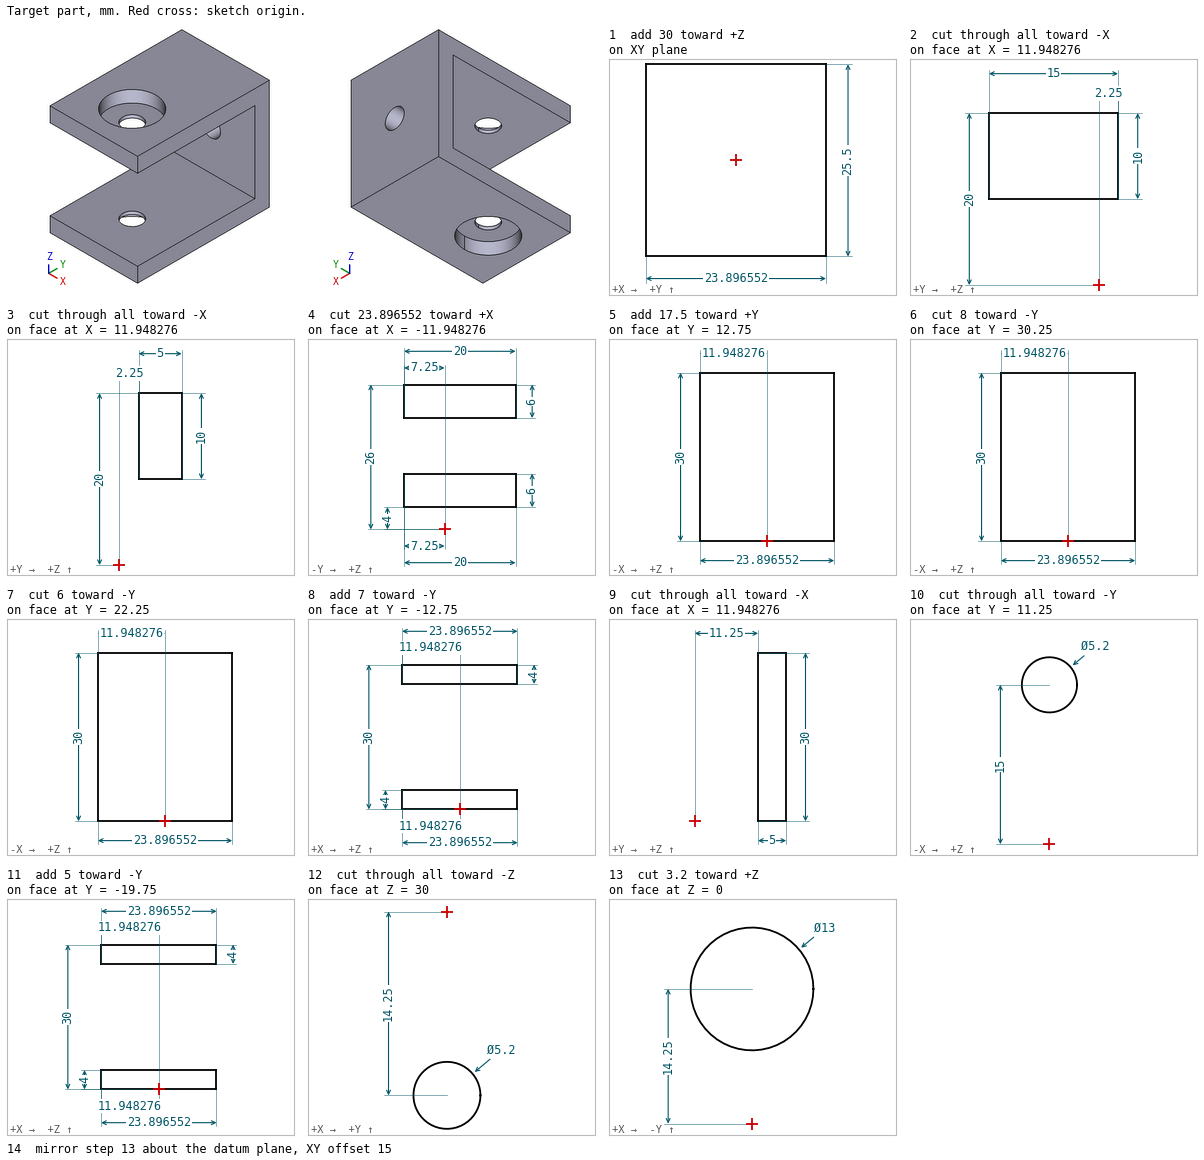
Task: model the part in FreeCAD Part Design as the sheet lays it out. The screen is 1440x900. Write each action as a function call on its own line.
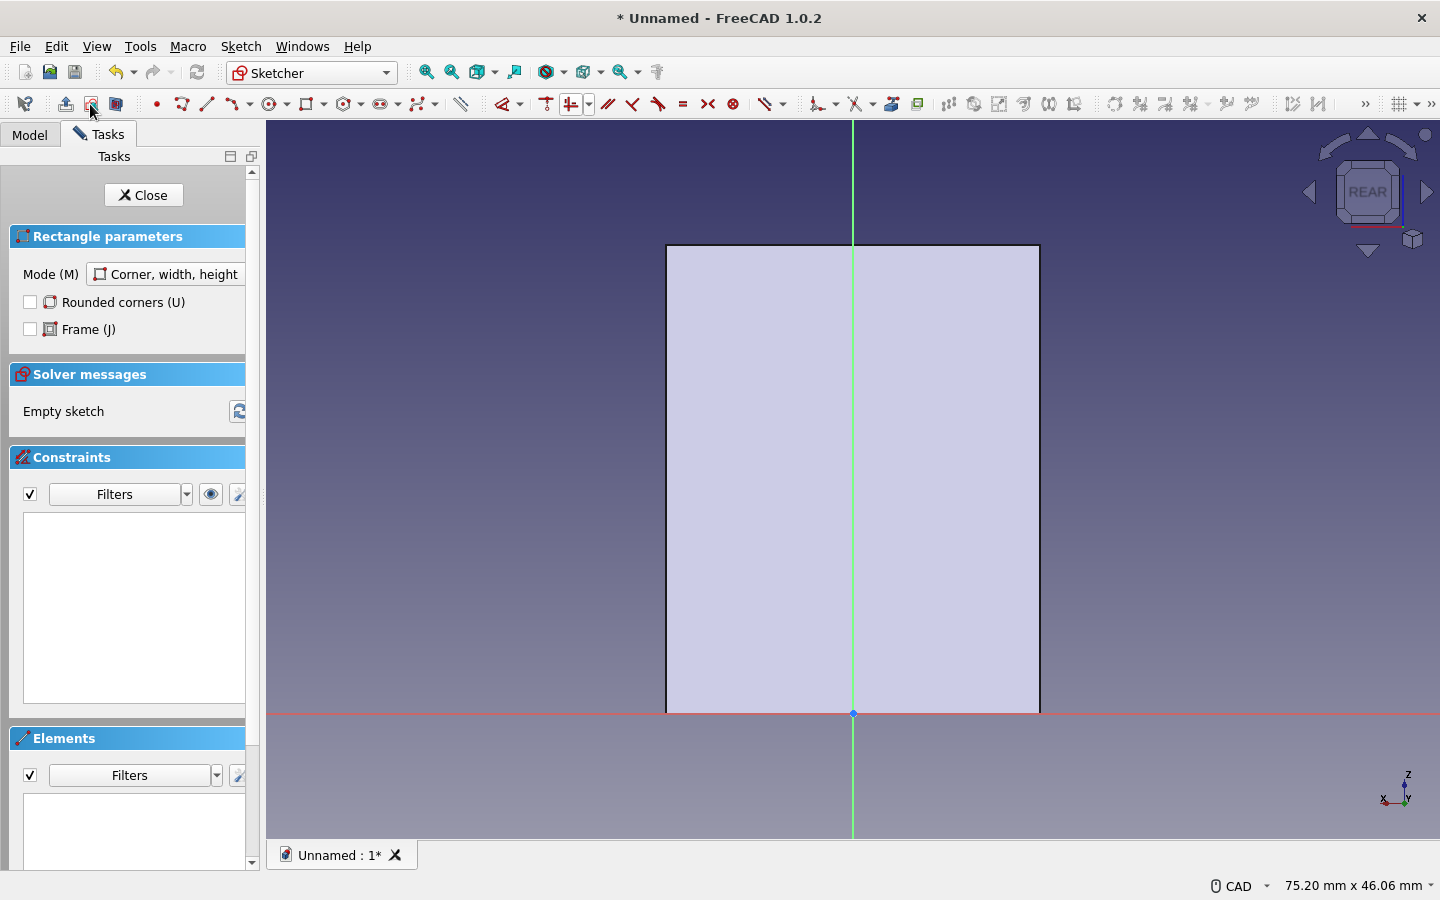
click(666, 245)
click(1040, 714)
key(Escape)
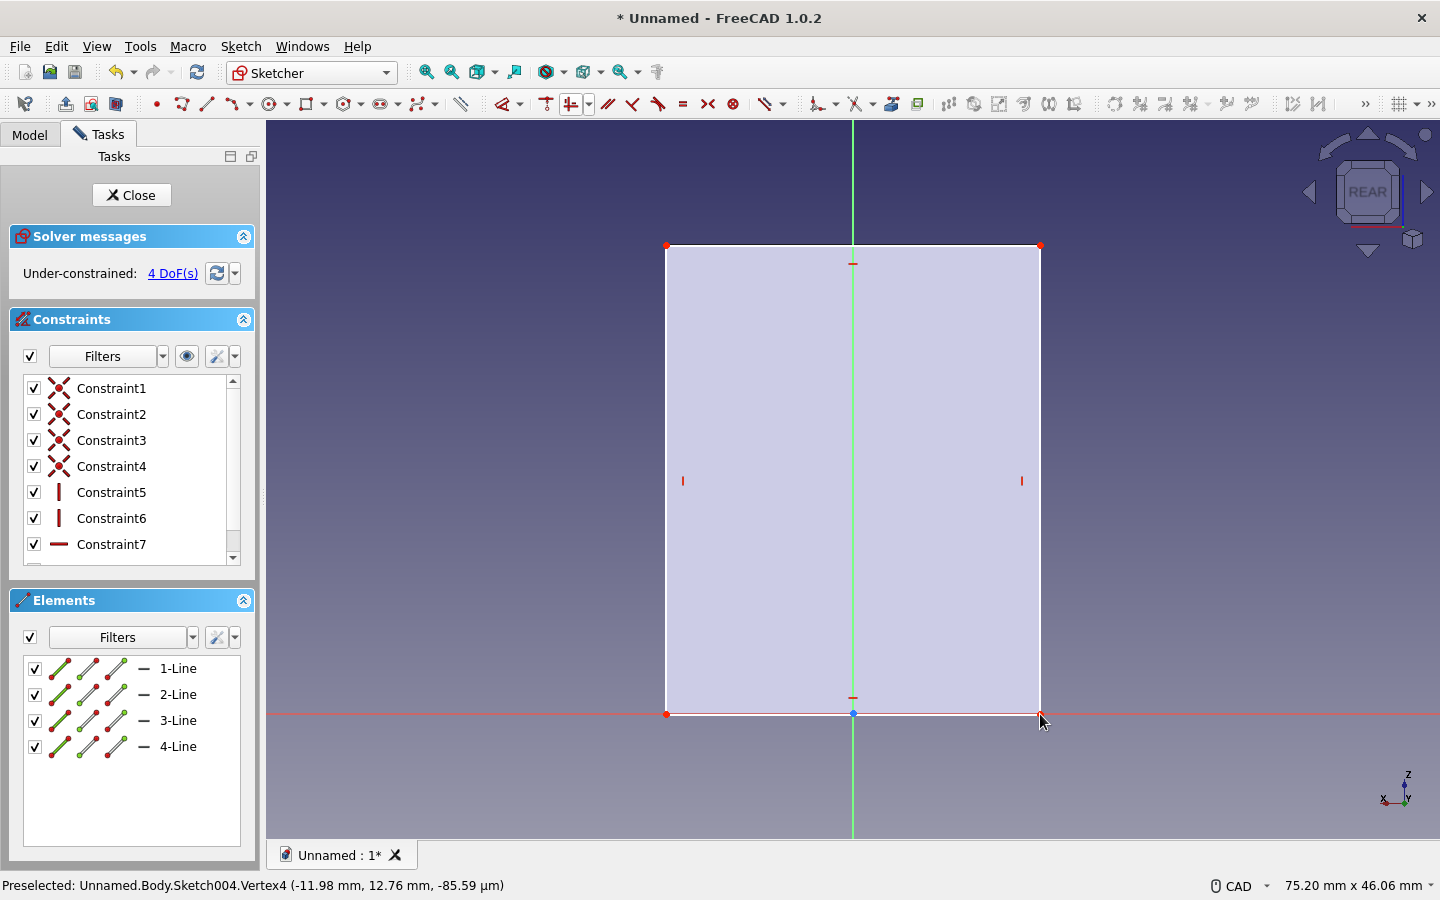
click(666, 715)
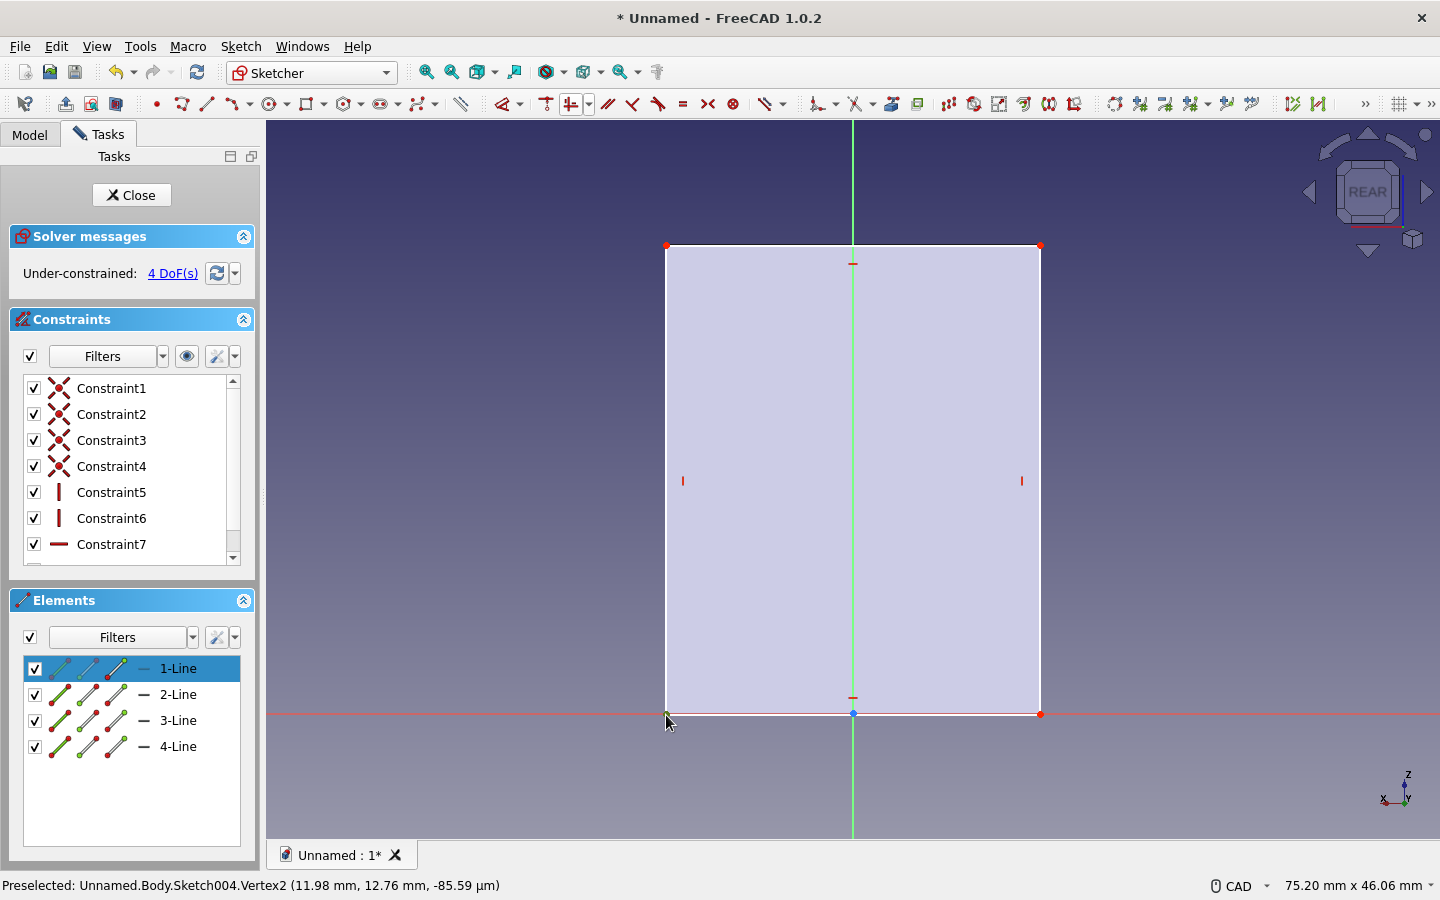
click(364, 714)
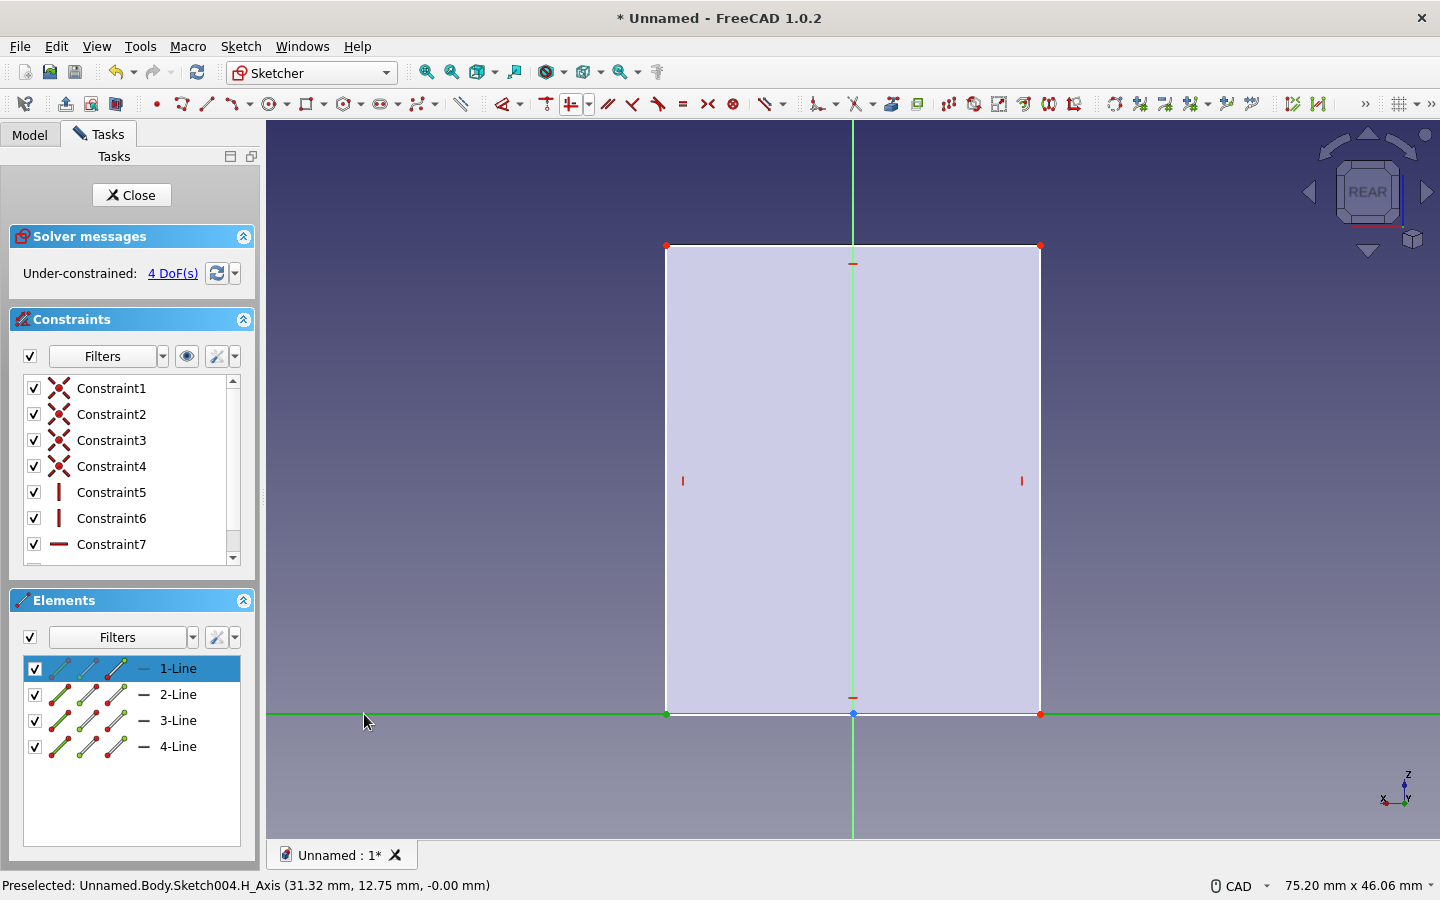
click(546, 104)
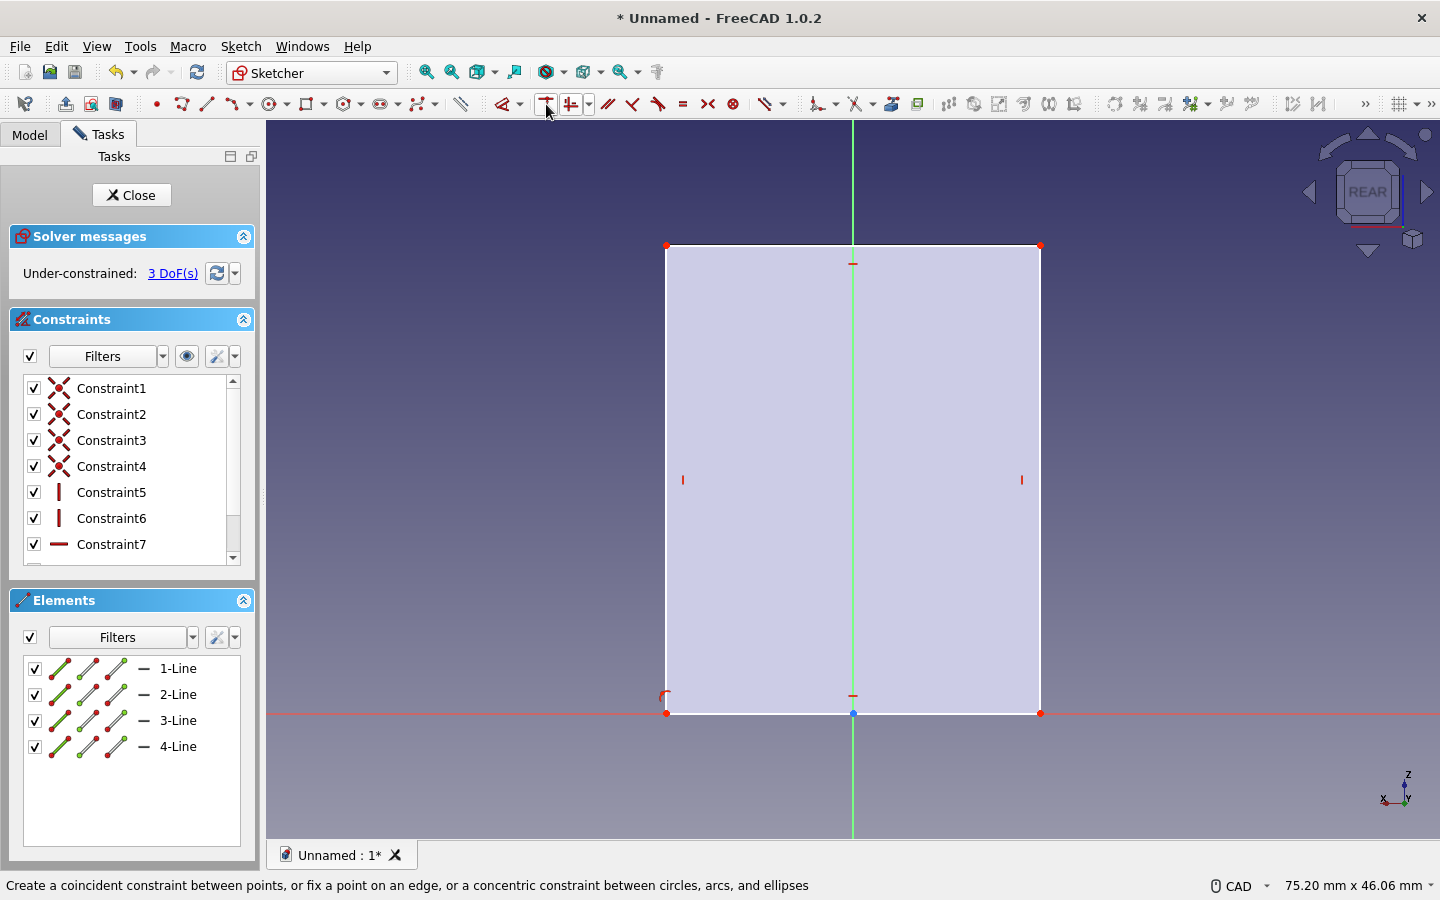
click(502, 104)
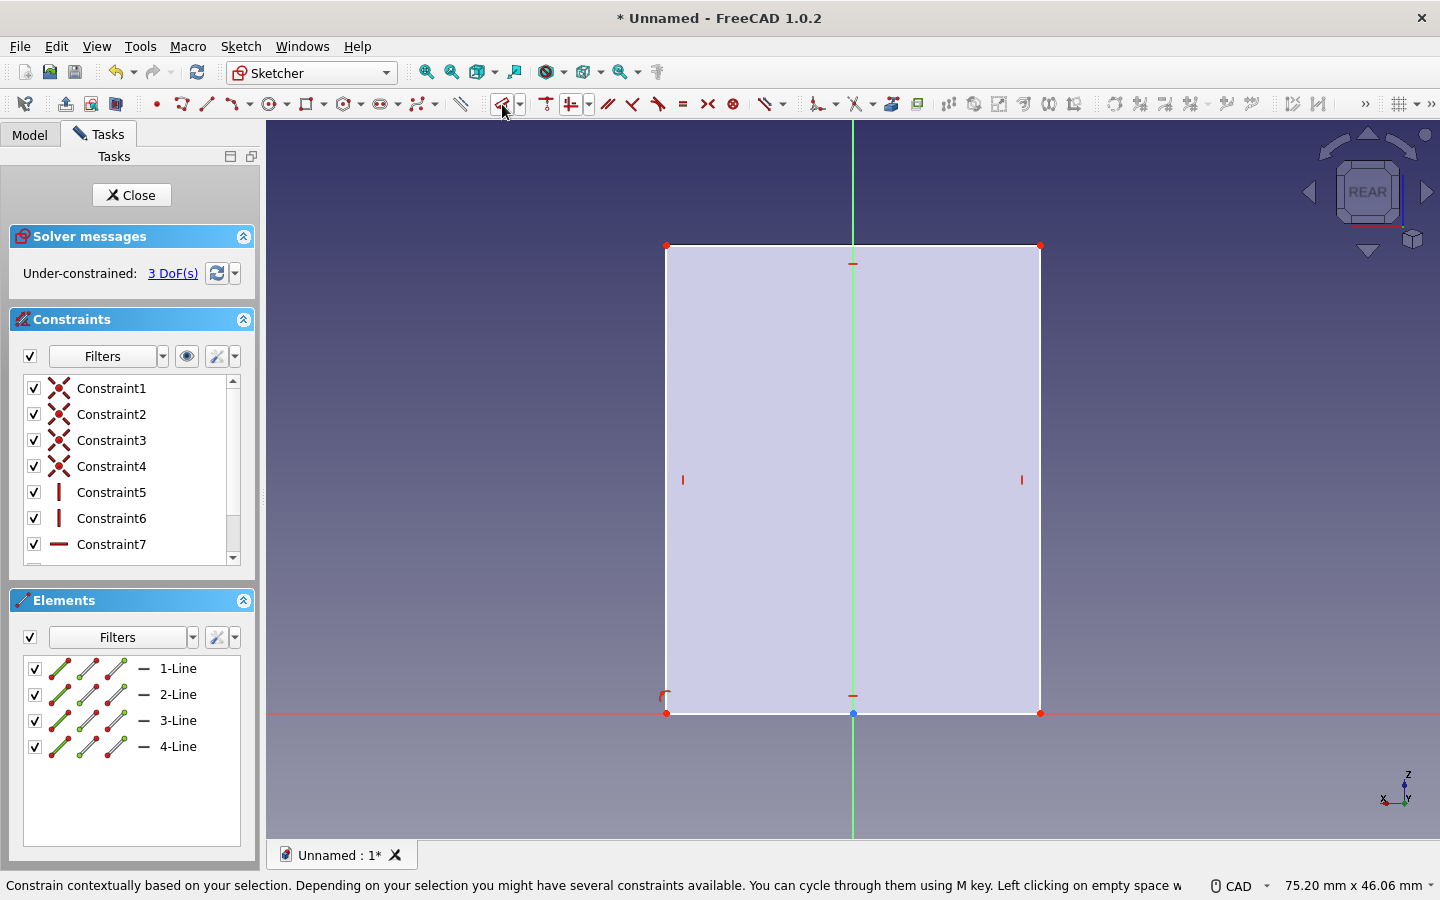
click(666, 386)
click(632, 480)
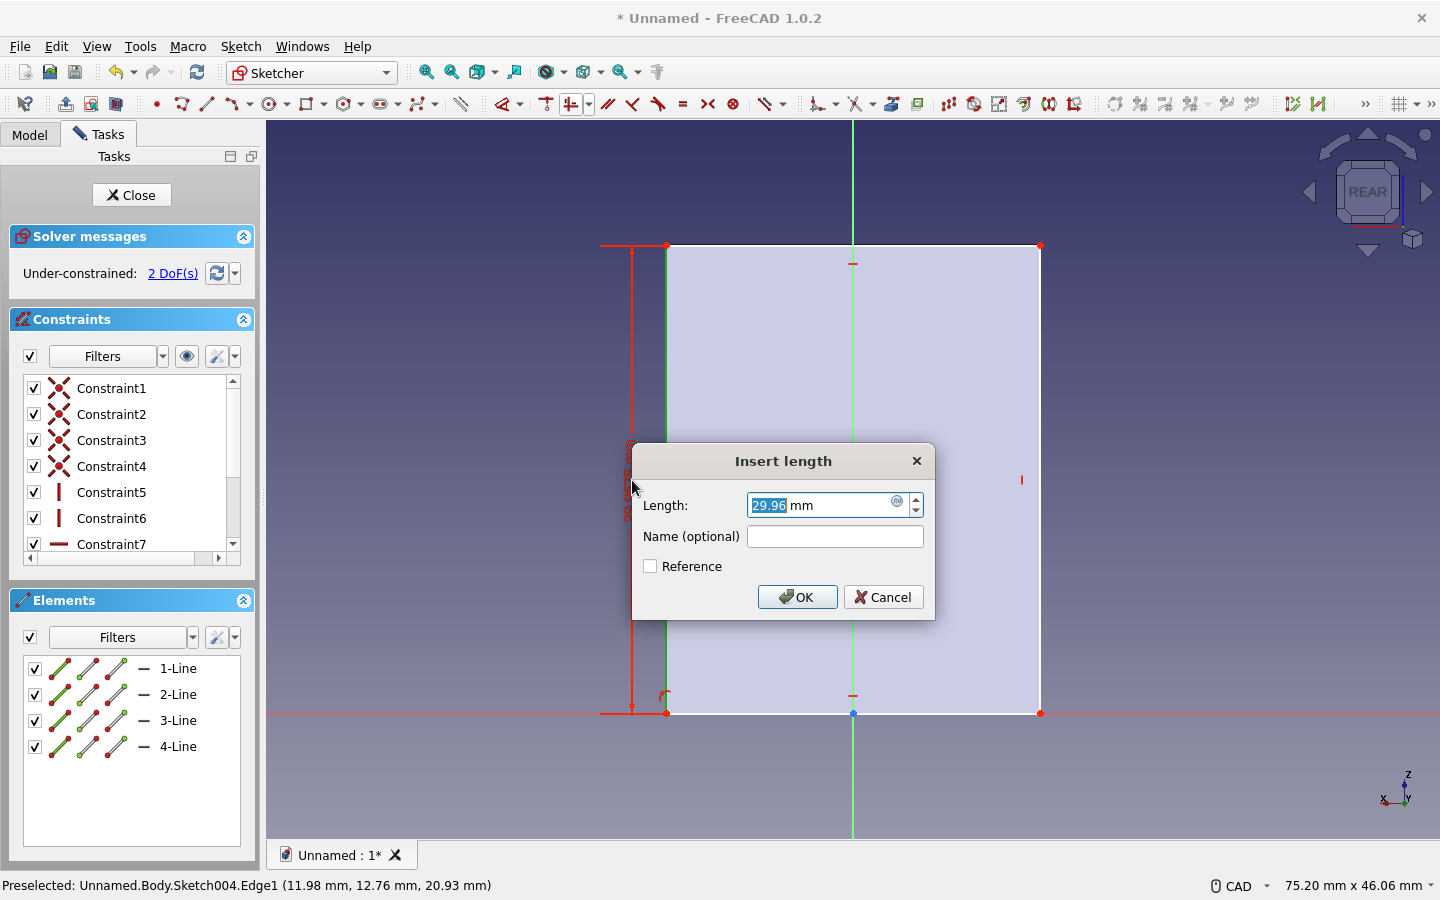
text(30)
key(Return)